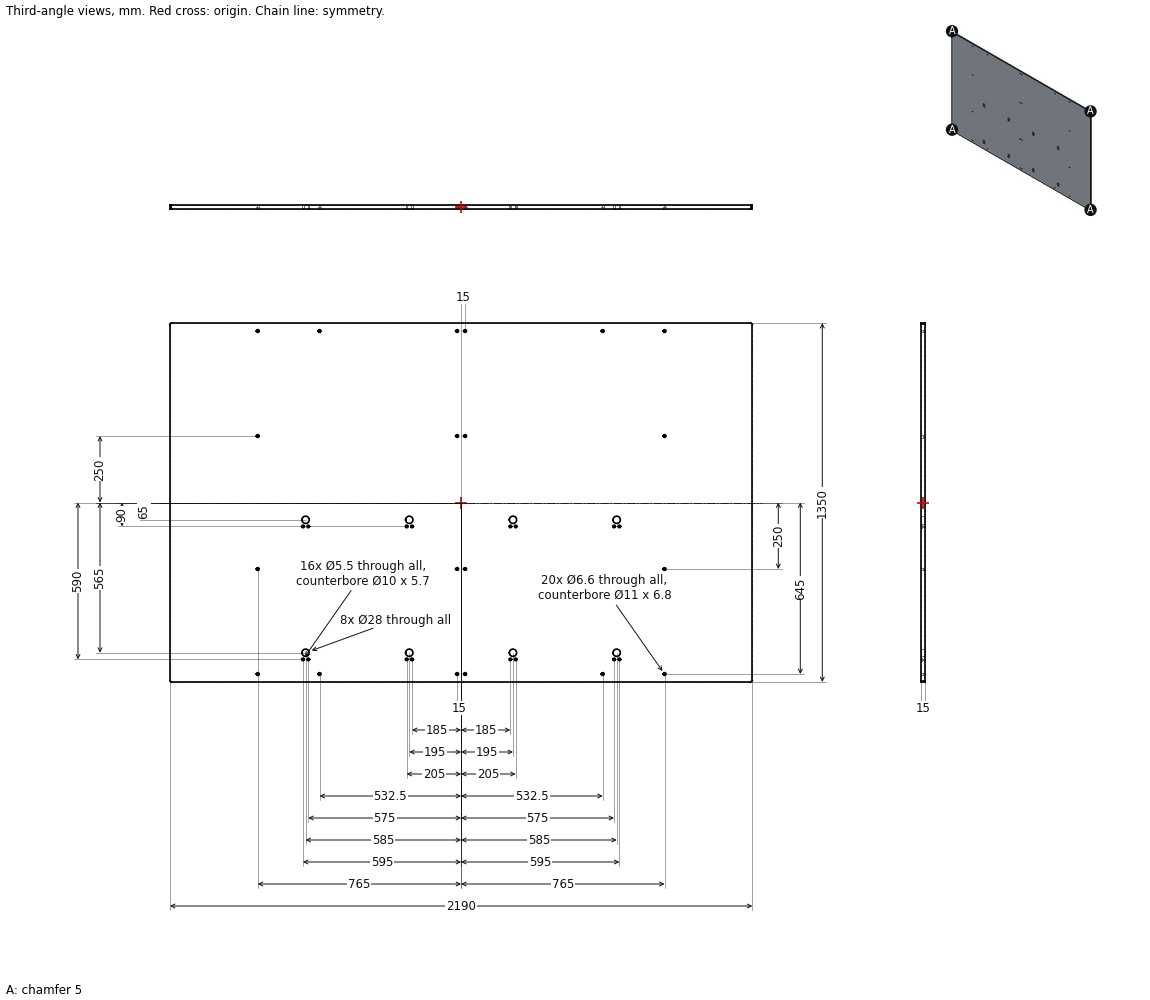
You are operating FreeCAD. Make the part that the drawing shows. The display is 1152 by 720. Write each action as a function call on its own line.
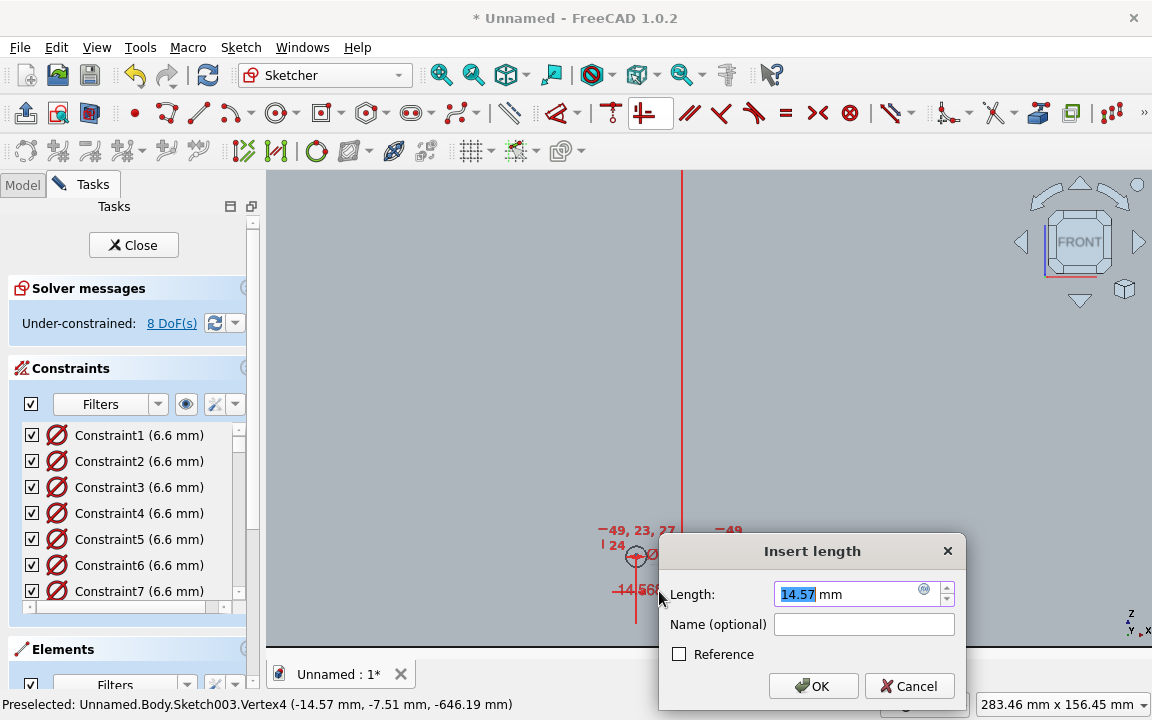
text(15)
key(Return)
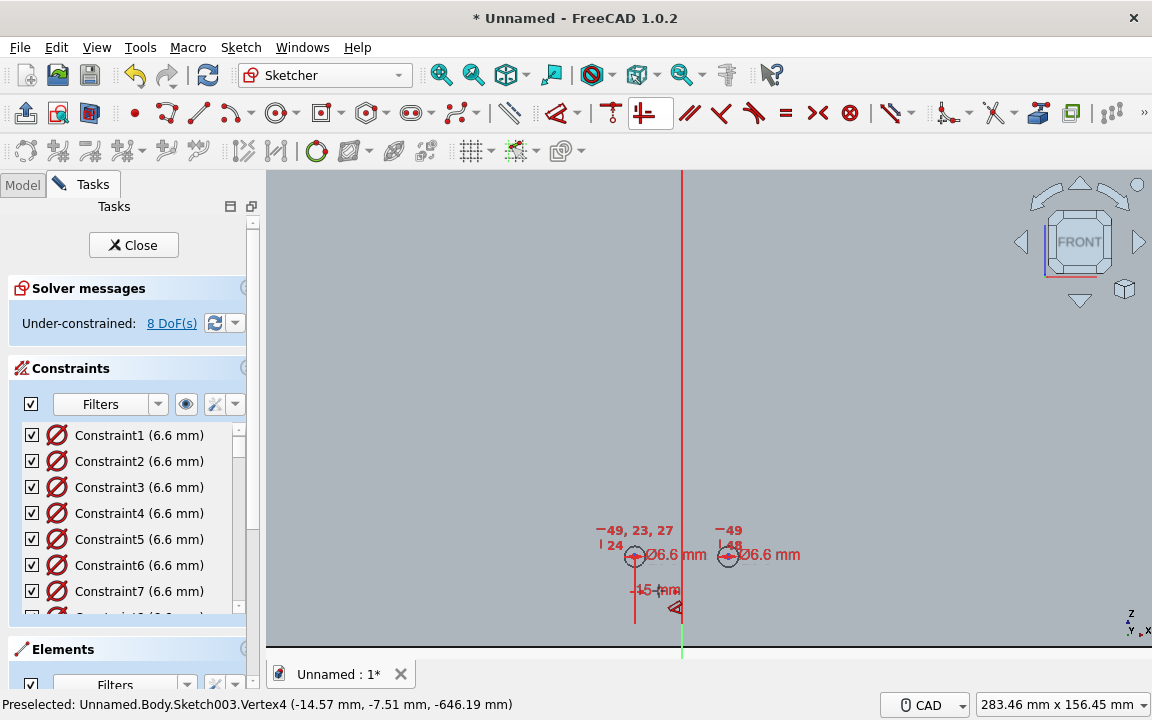
scroll(637, 565, down, 13)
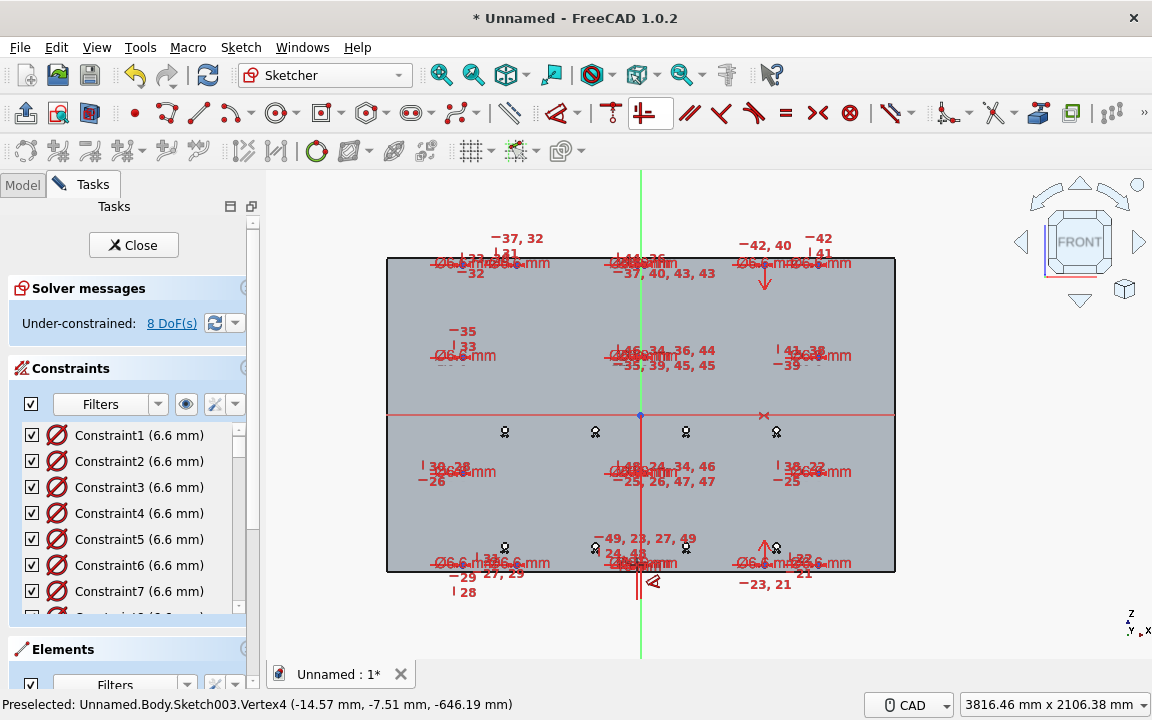
scroll(644, 265, up, 13)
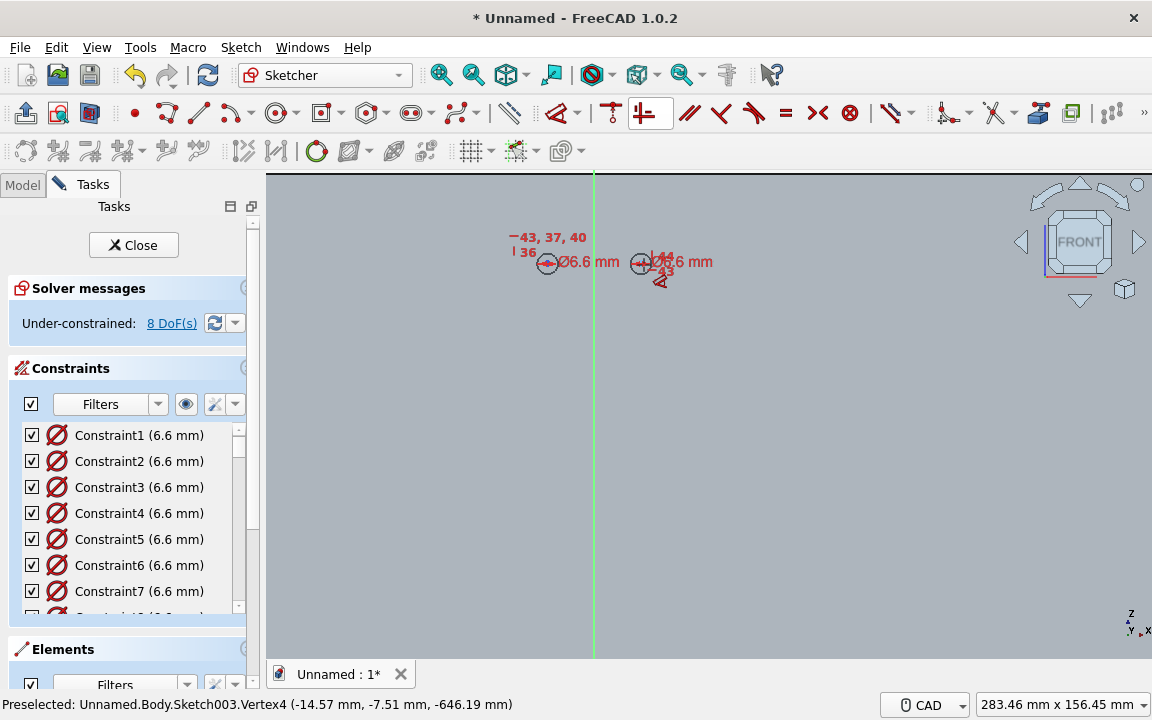
click(641, 264)
click(618, 230)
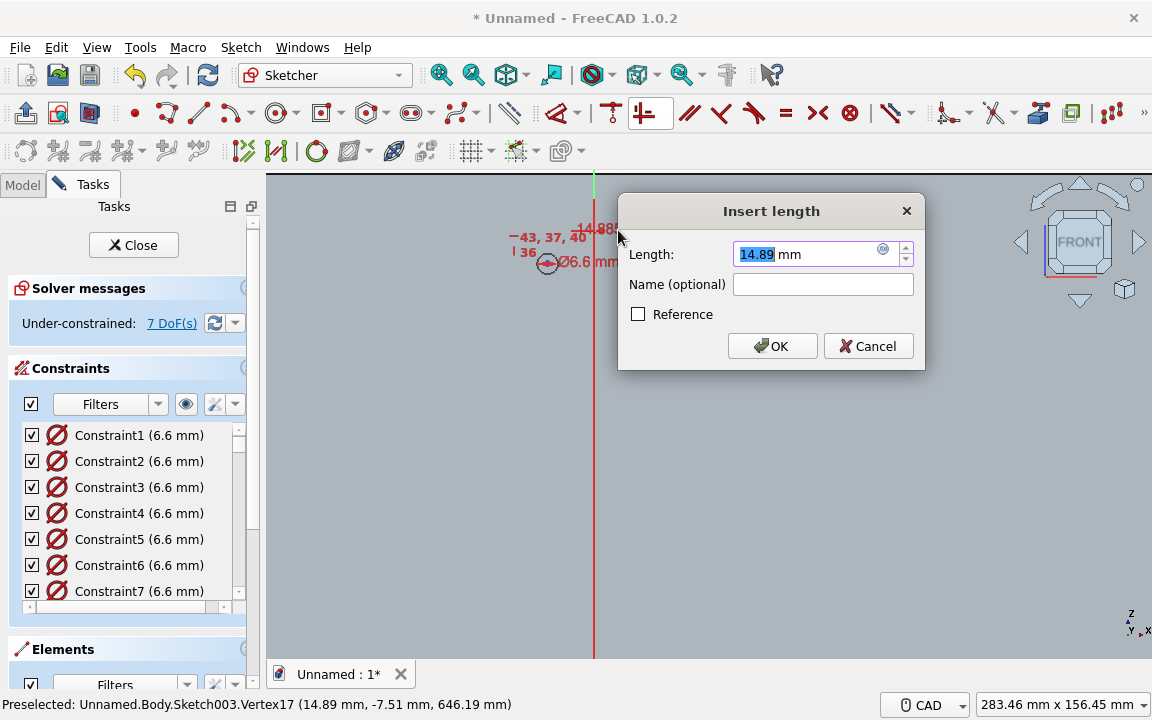
text(15)
key(Return)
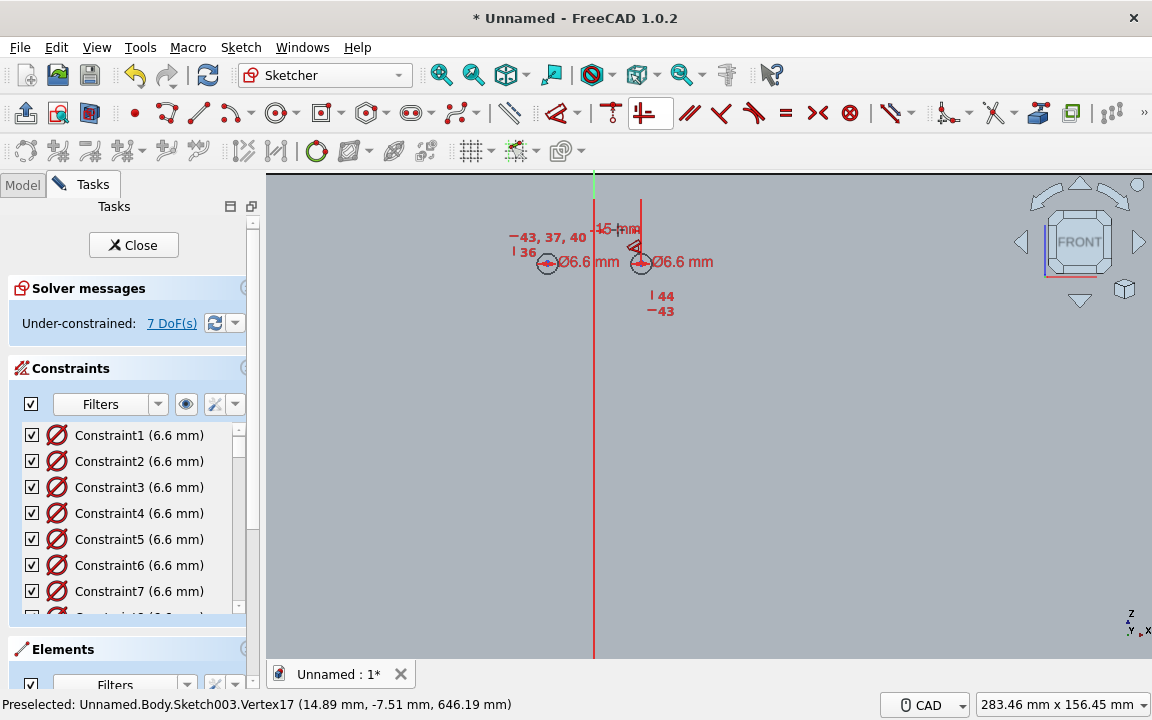
scroll(644, 265, down, 13)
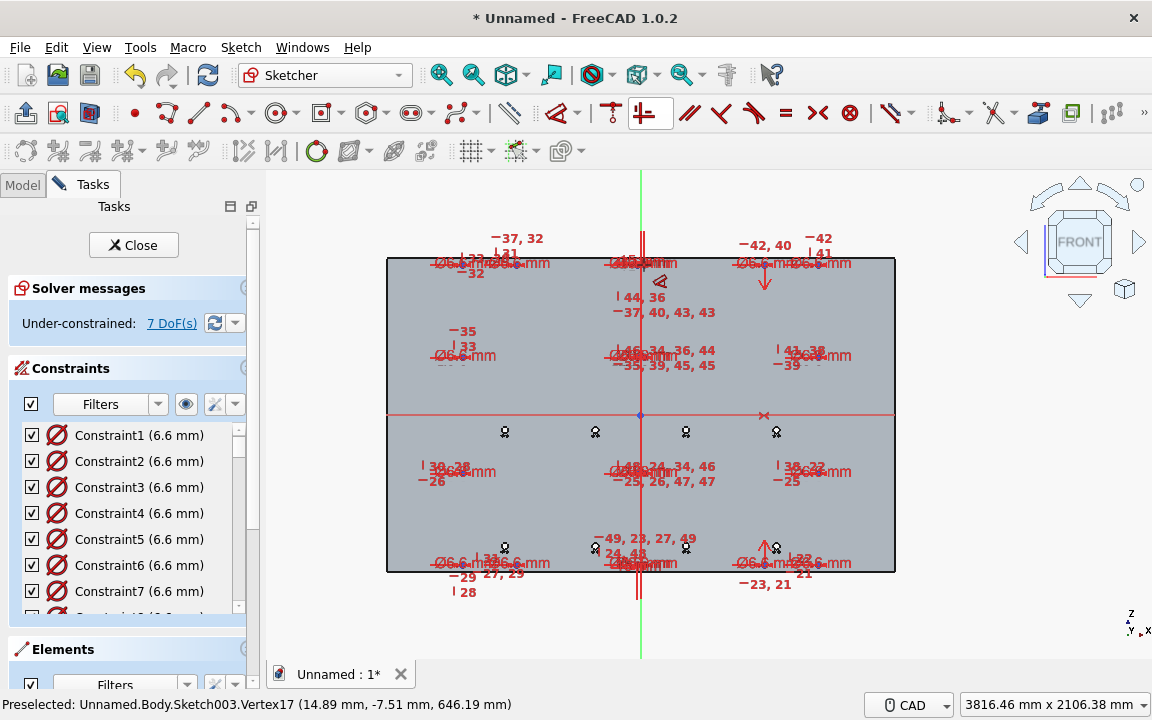
click(818, 565)
click(729, 599)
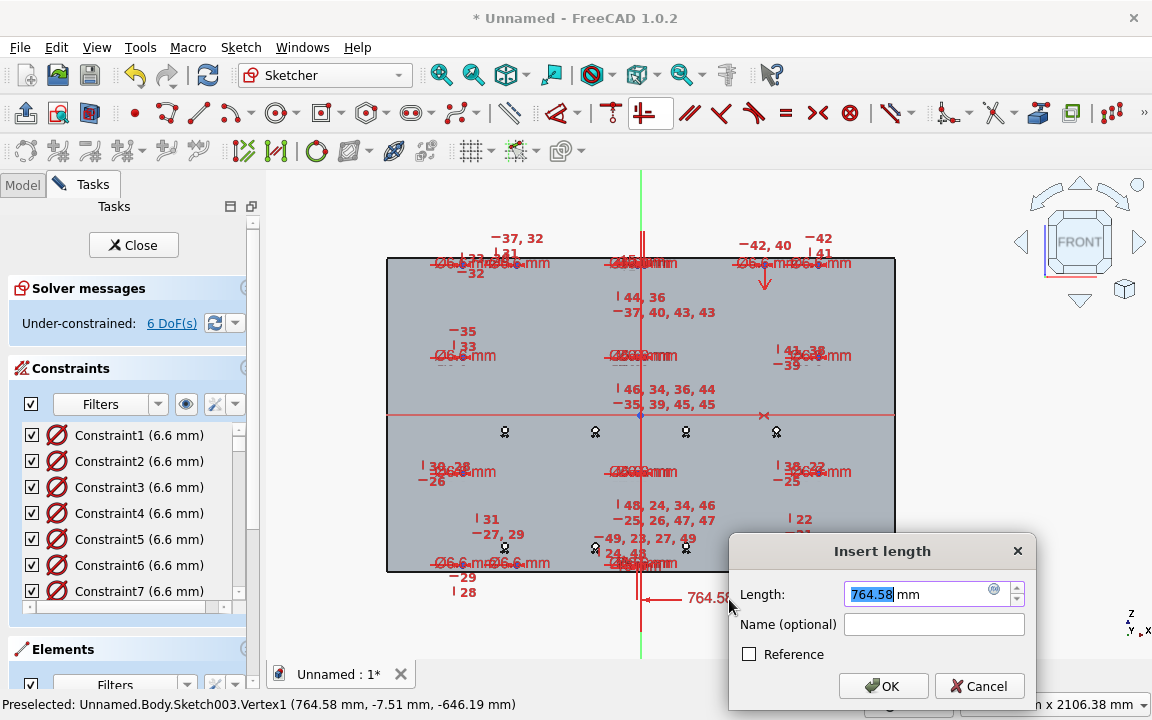
text(765)
key(Return)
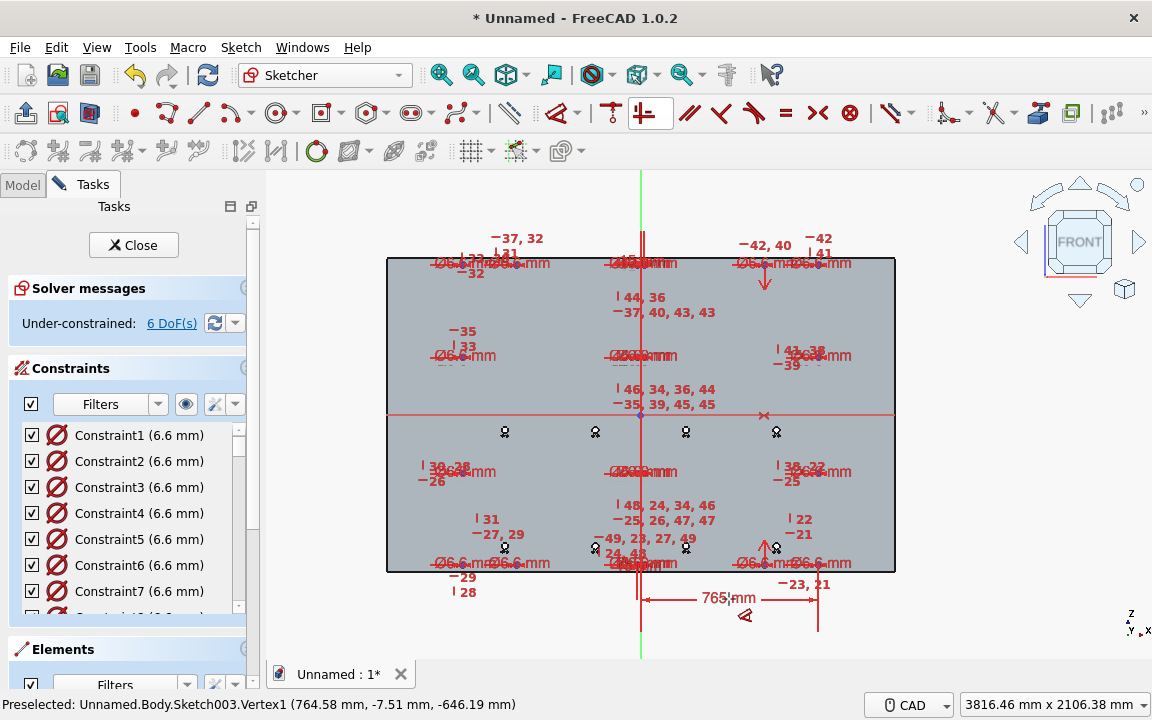
click(818, 565)
click(852, 490)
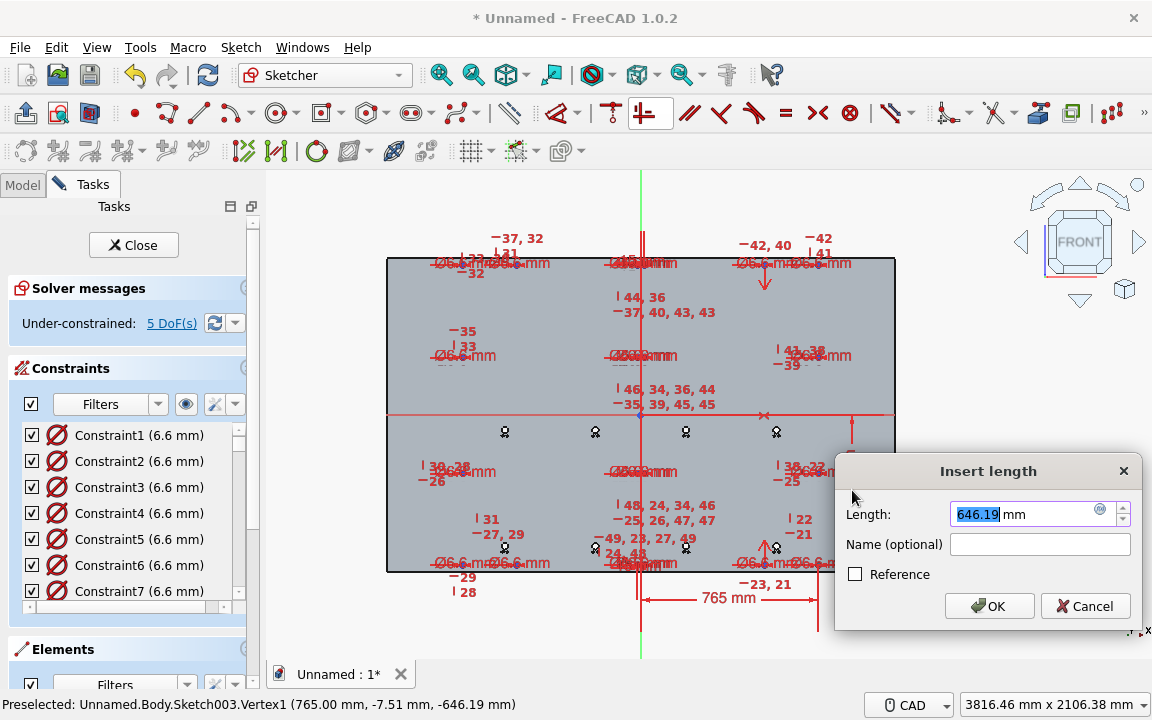
text(645)
key(Return)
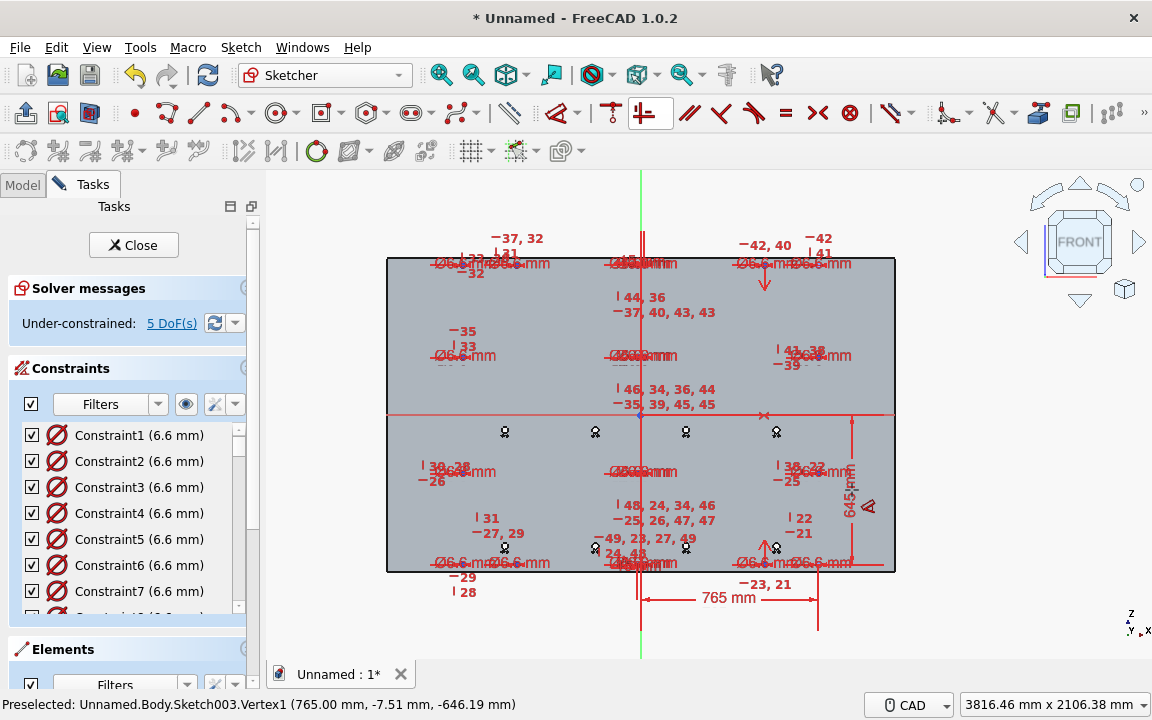
click(818, 474)
click(852, 444)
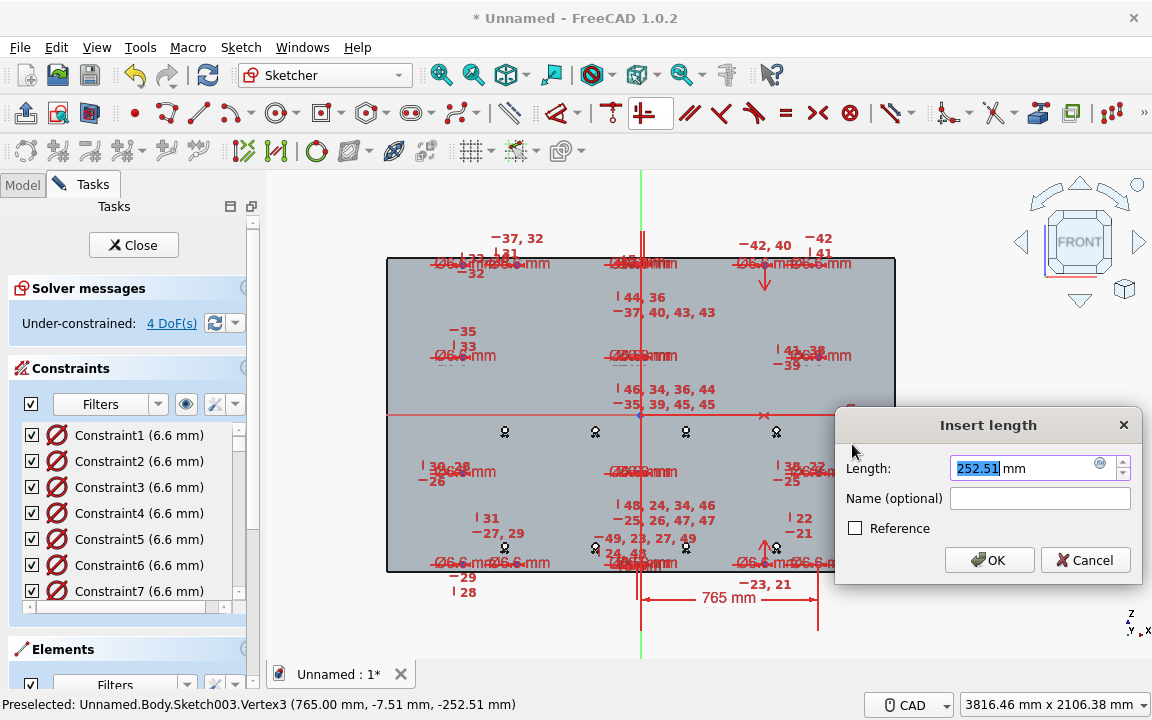
text(250)
key(Return)